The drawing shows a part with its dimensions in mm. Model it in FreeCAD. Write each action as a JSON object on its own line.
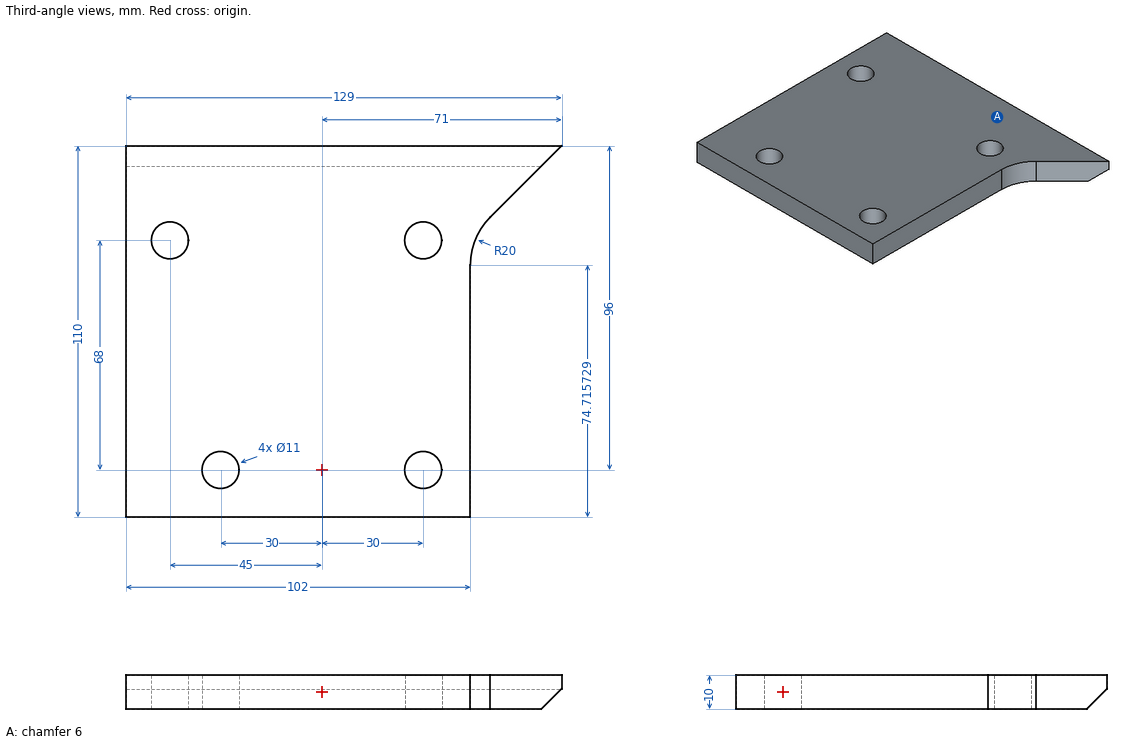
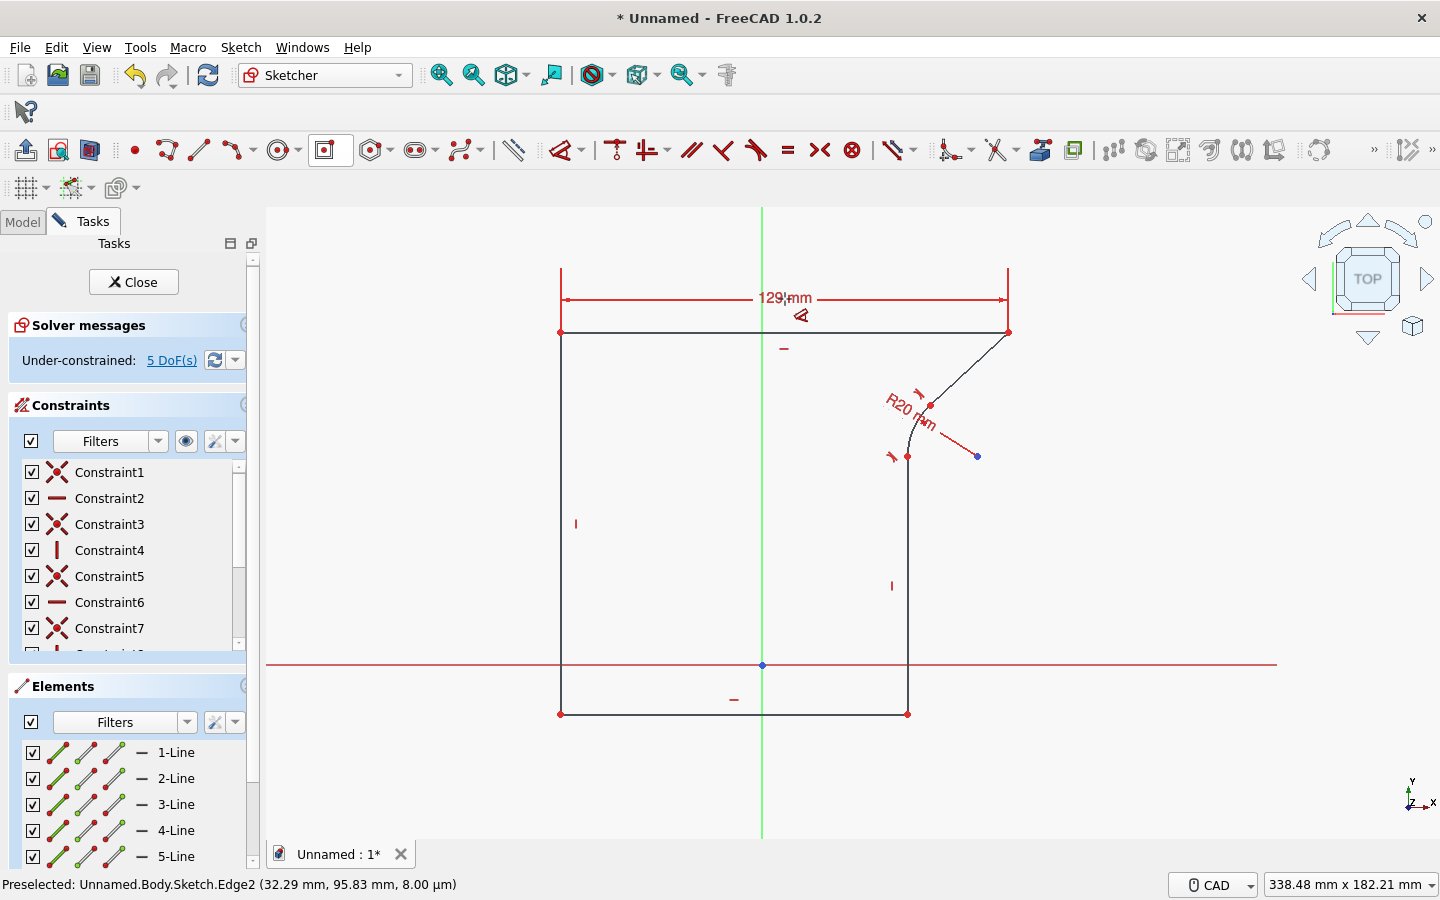
{"action": "left_click", "coordinate": [561, 448]}
{"action": "left_click", "coordinate": [527, 524]}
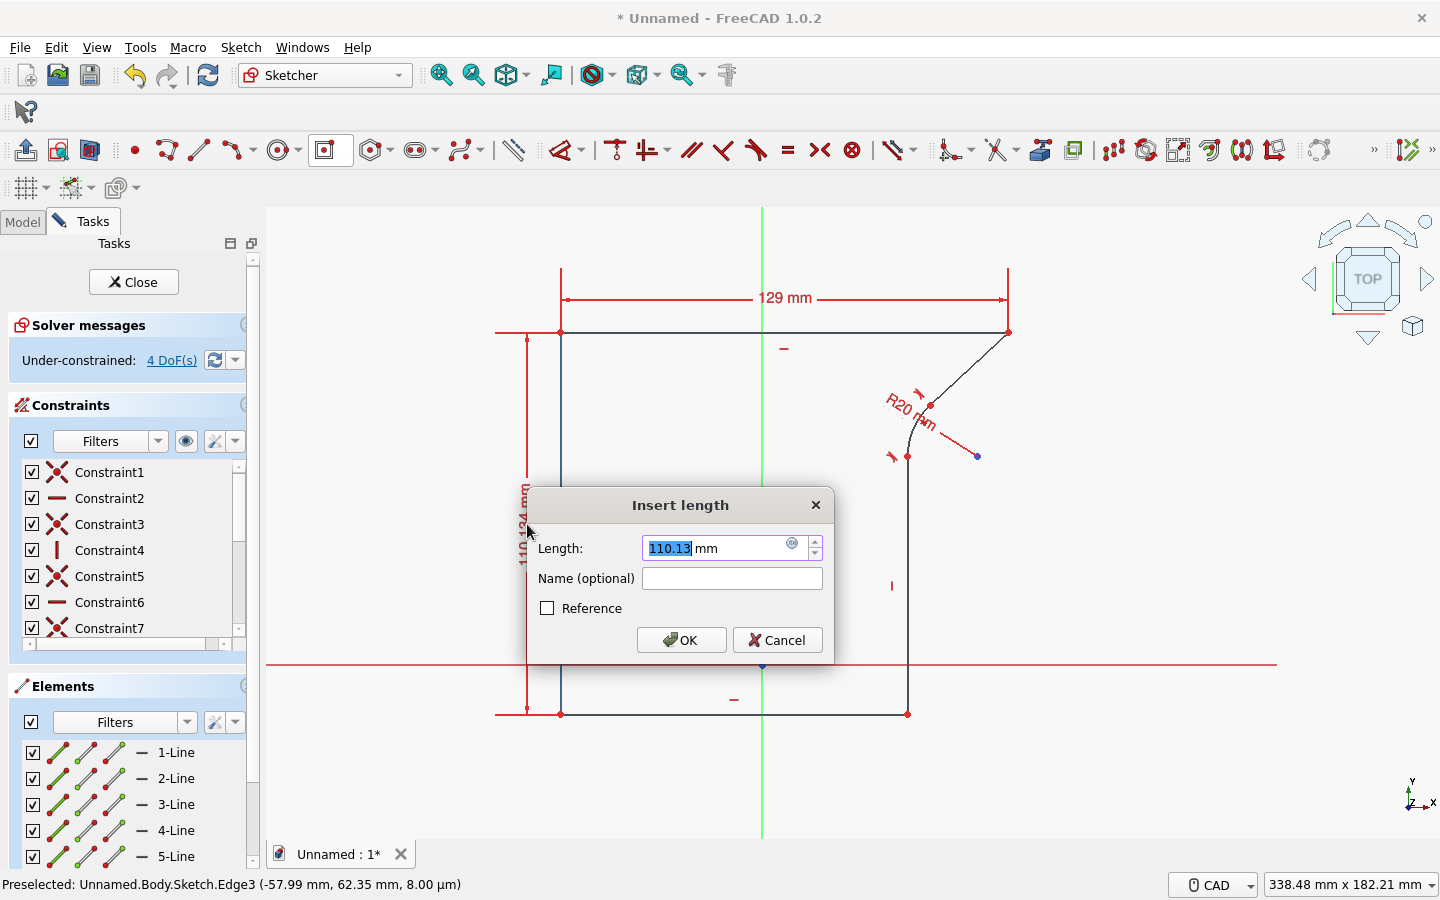
{"action": "type", "text": "110"}
{"action": "key", "text": "Return"}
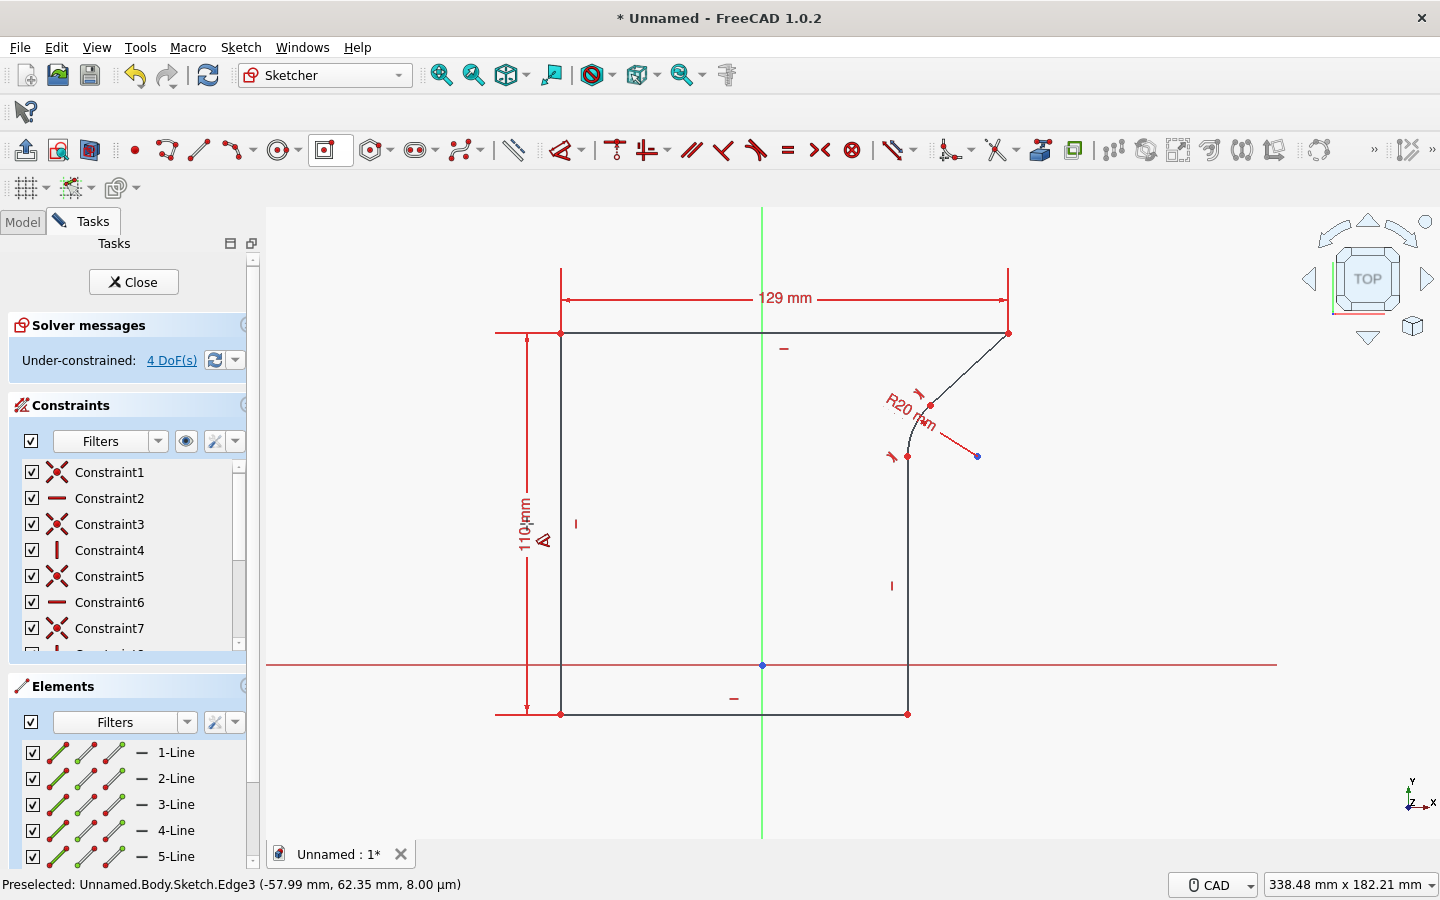
{"action": "left_click", "coordinate": [665, 715]}
{"action": "left_click", "coordinate": [734, 749]}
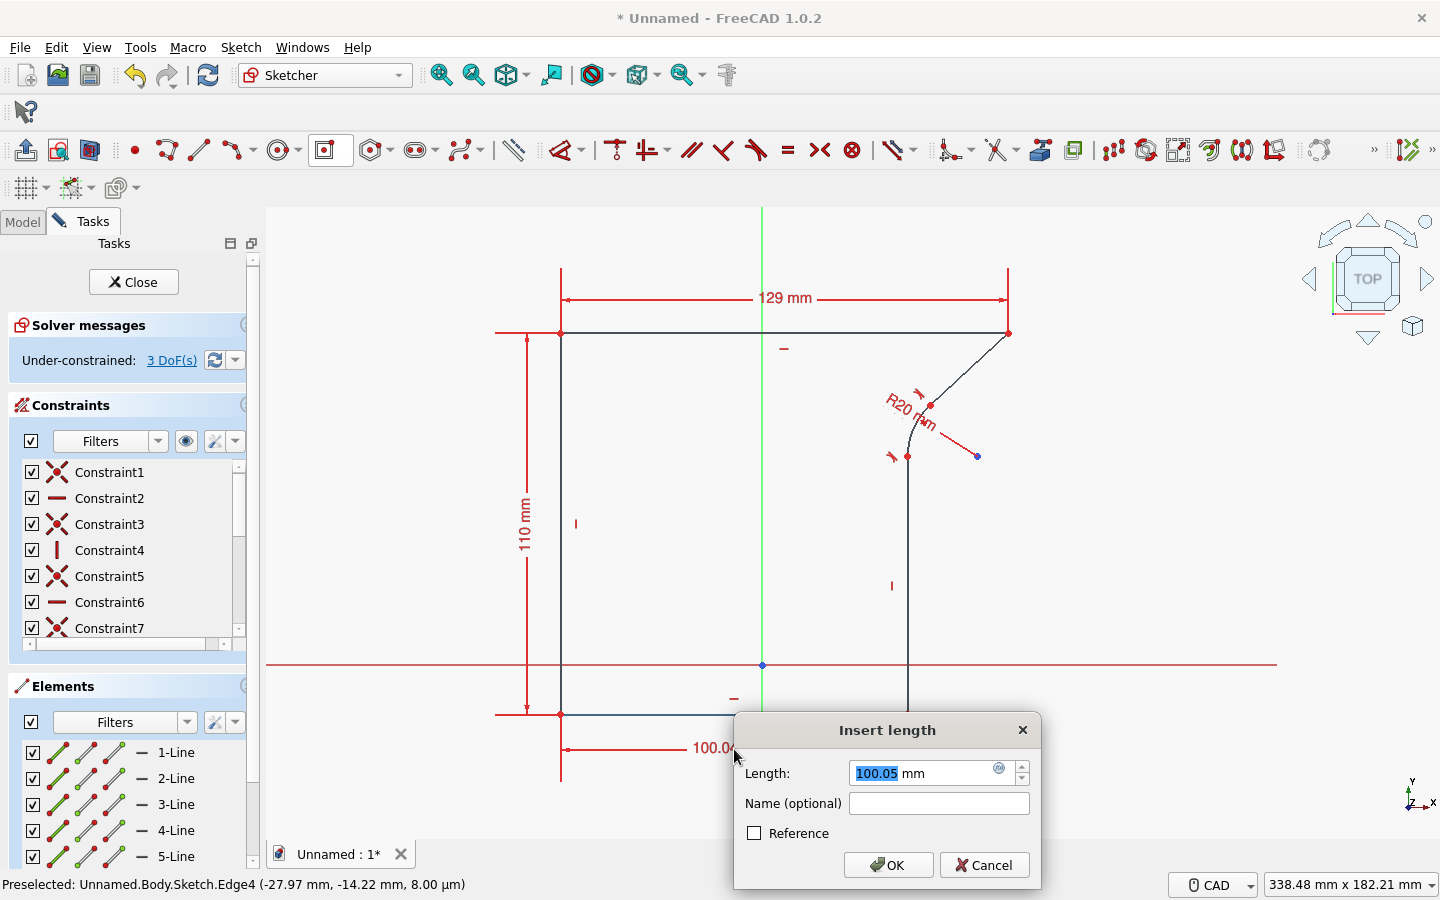
{"action": "type", "text": "102"}
{"action": "key", "text": "Return"}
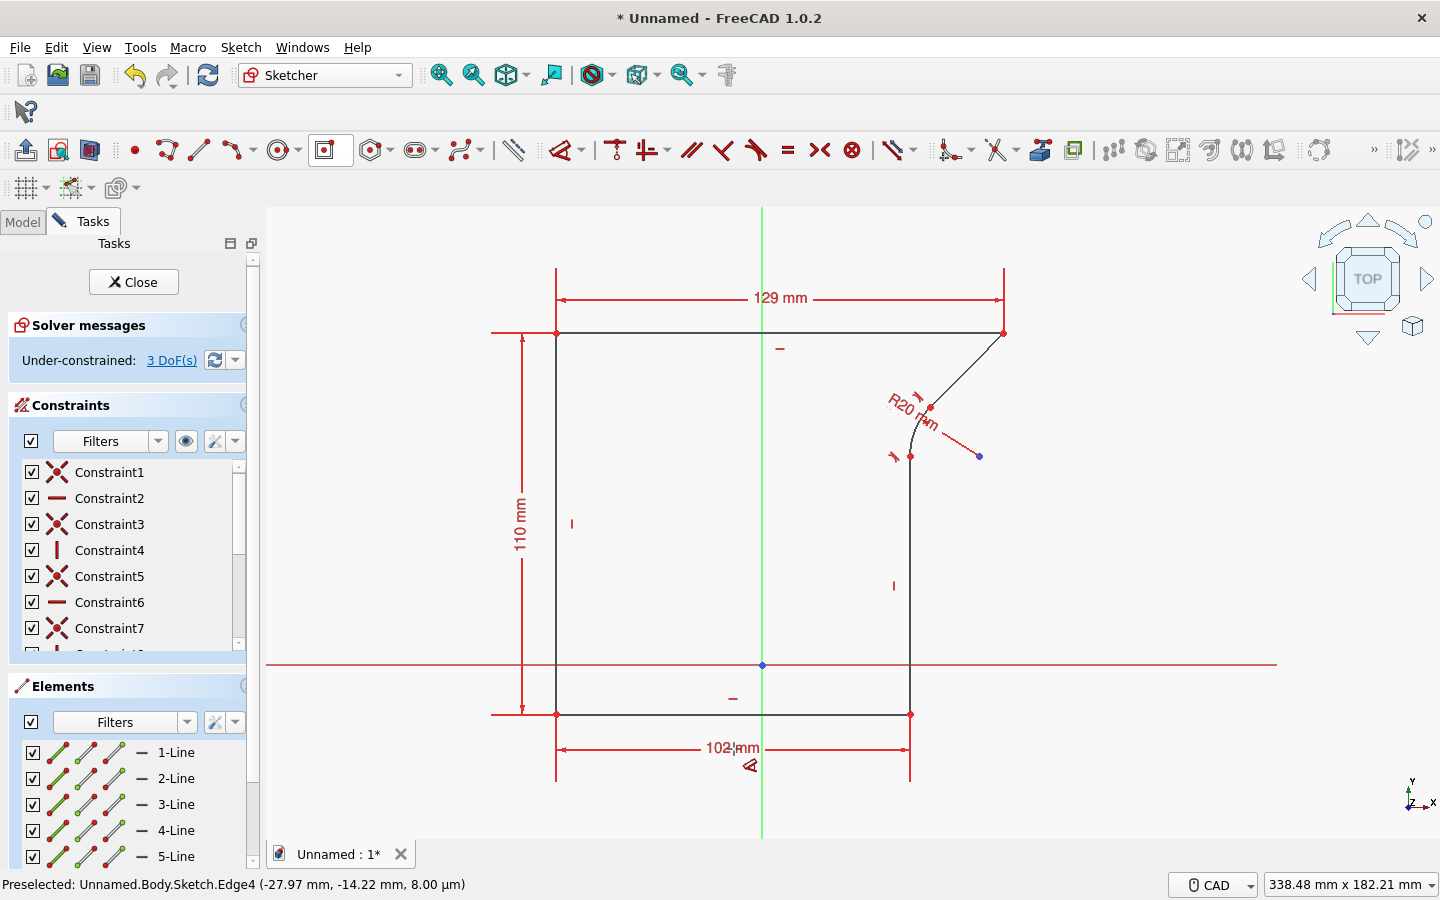
{"action": "left_click", "coordinate": [1004, 333]}
{"action": "left_click", "coordinate": [883, 299]}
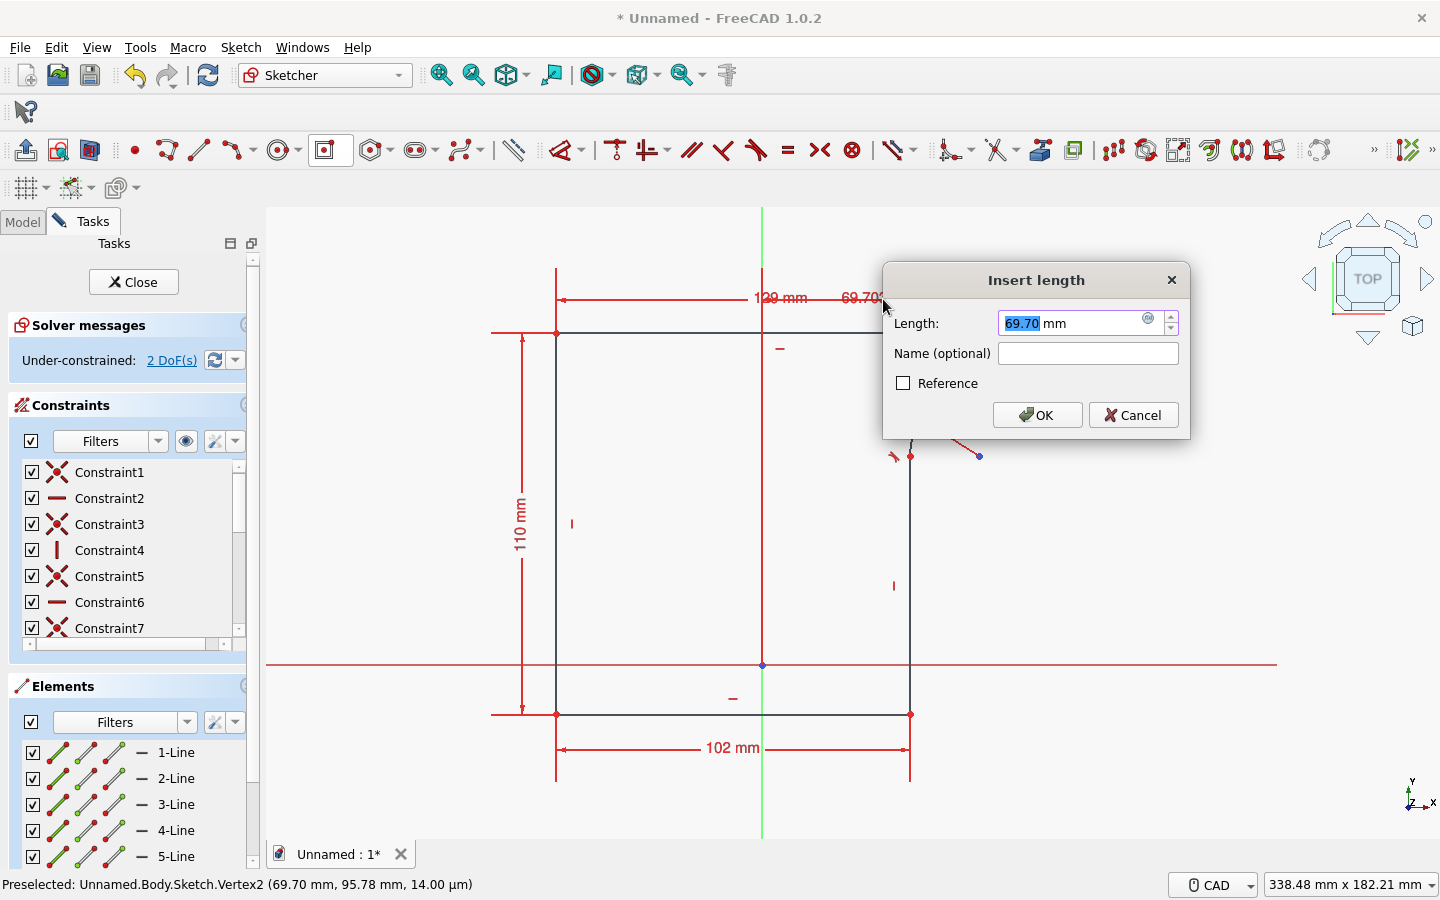
{"action": "type", "text": "71"}
{"action": "key", "text": "Return"}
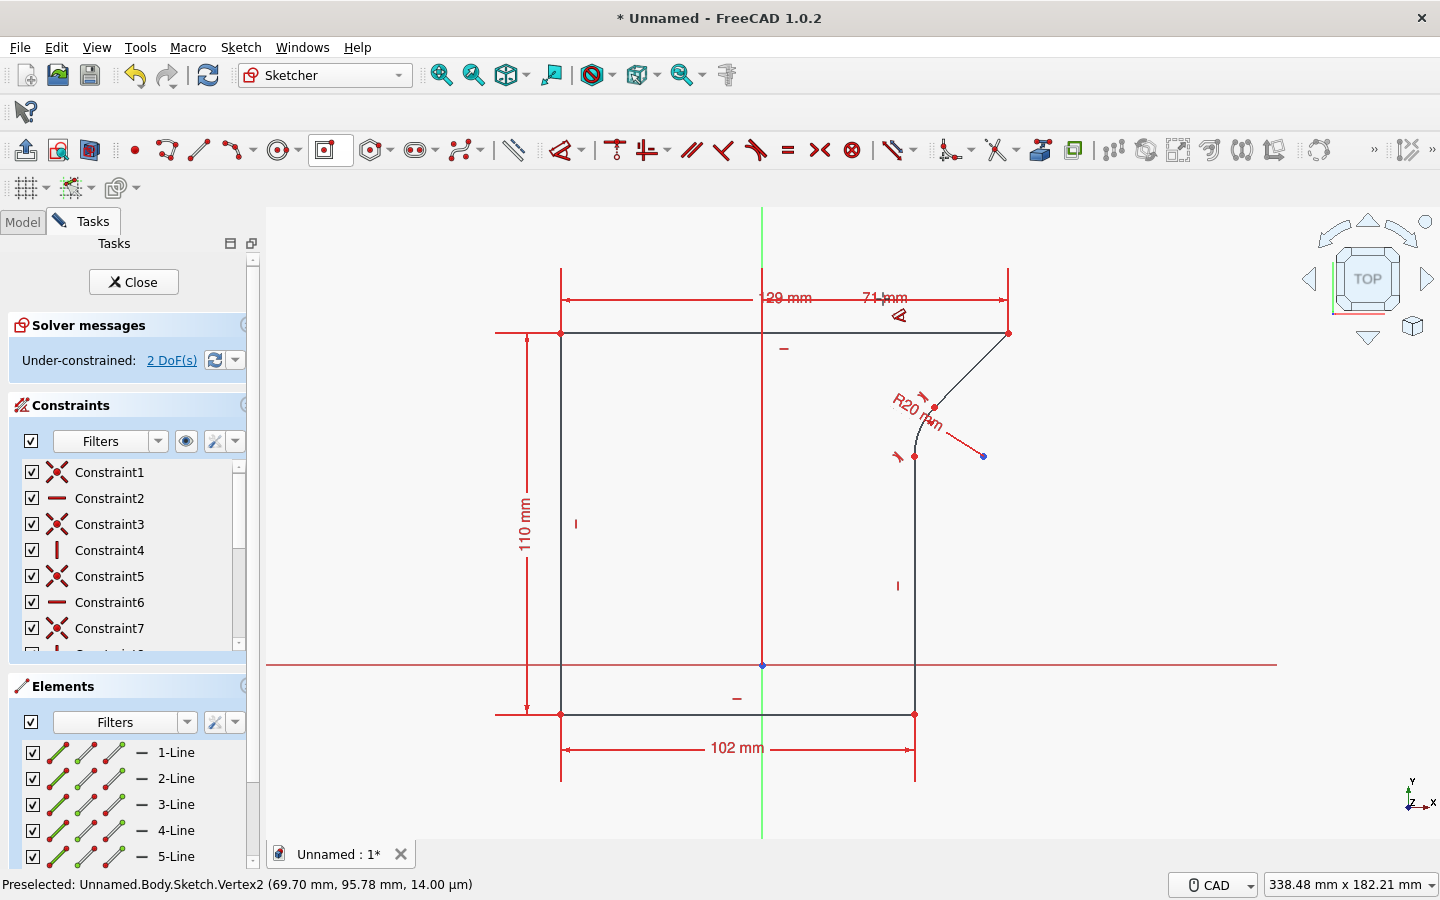
{"action": "left_click", "coordinate": [1008, 333]}
{"action": "left_click", "coordinate": [1042, 499]}